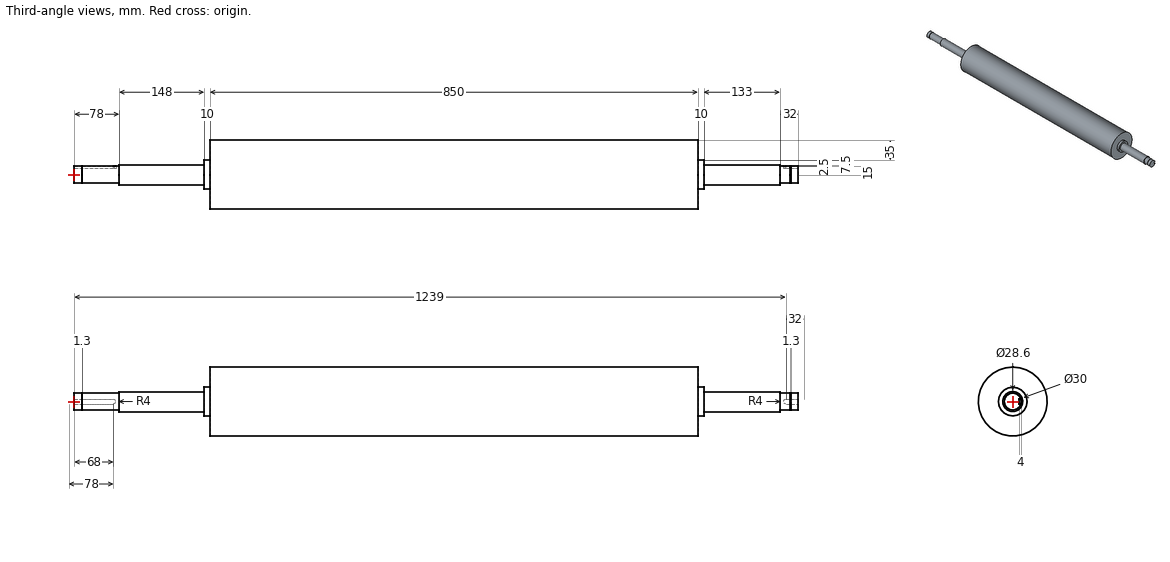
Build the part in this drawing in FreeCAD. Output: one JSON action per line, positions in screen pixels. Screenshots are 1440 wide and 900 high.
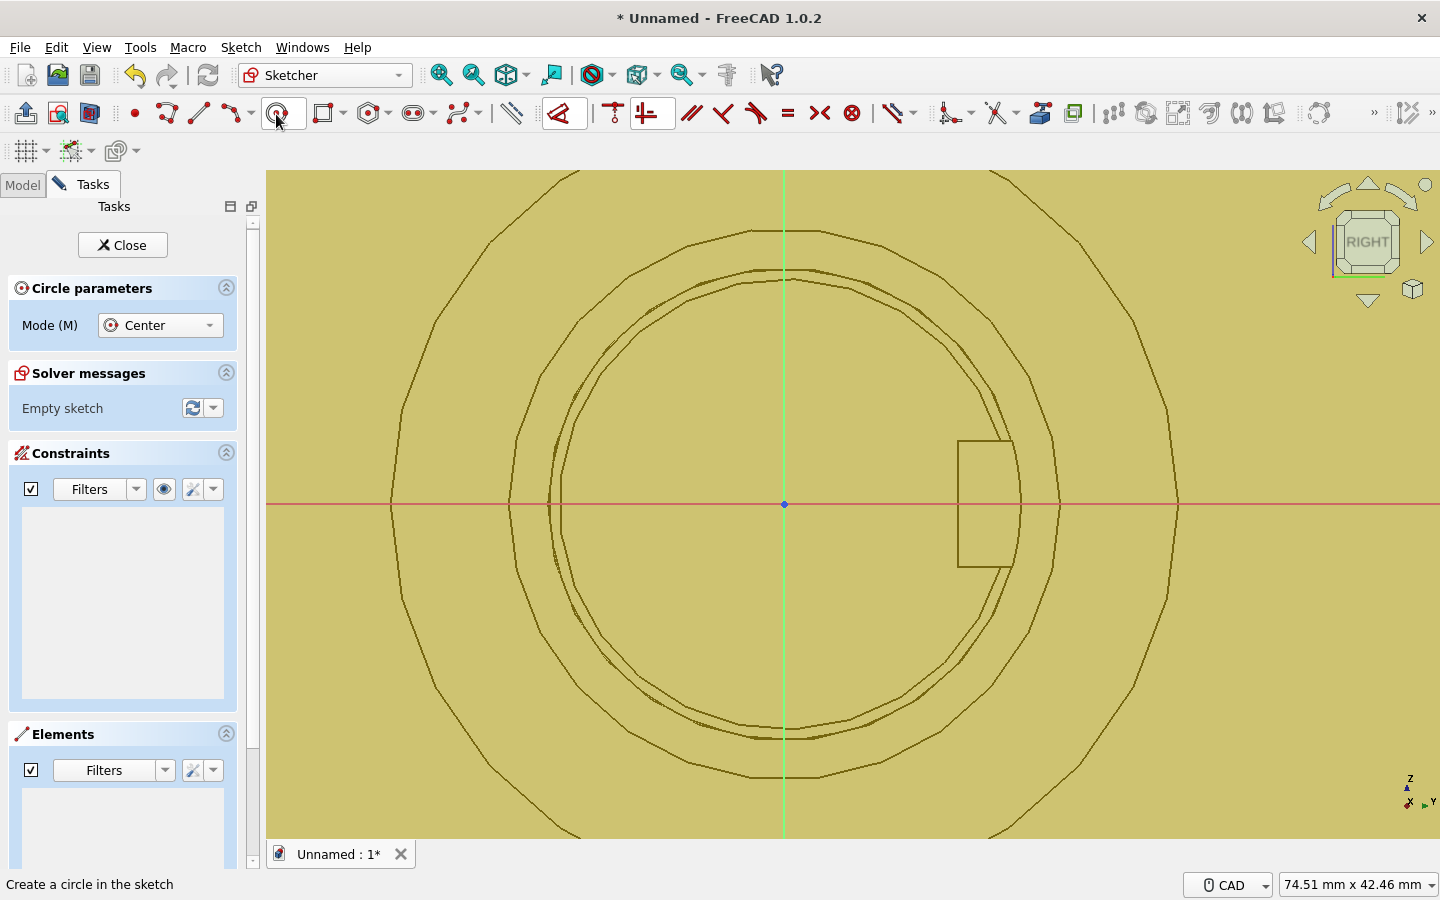
{"action": "left_click", "coordinate": [784, 504]}
{"action": "mouse_move", "coordinate": [952, 337]}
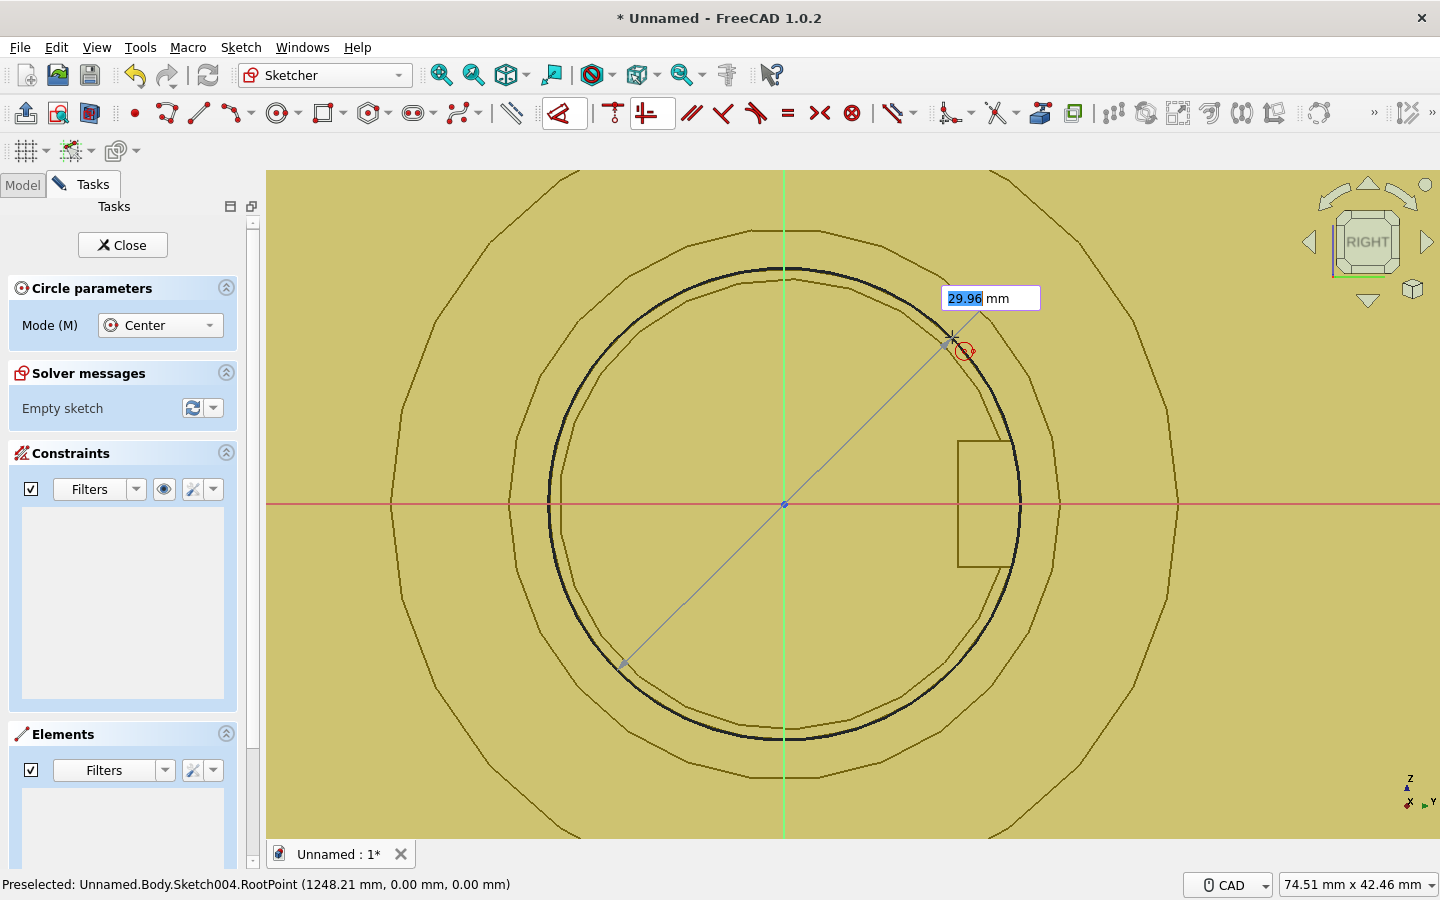
{"action": "type", "text": "30"}
{"action": "key", "text": "Return"}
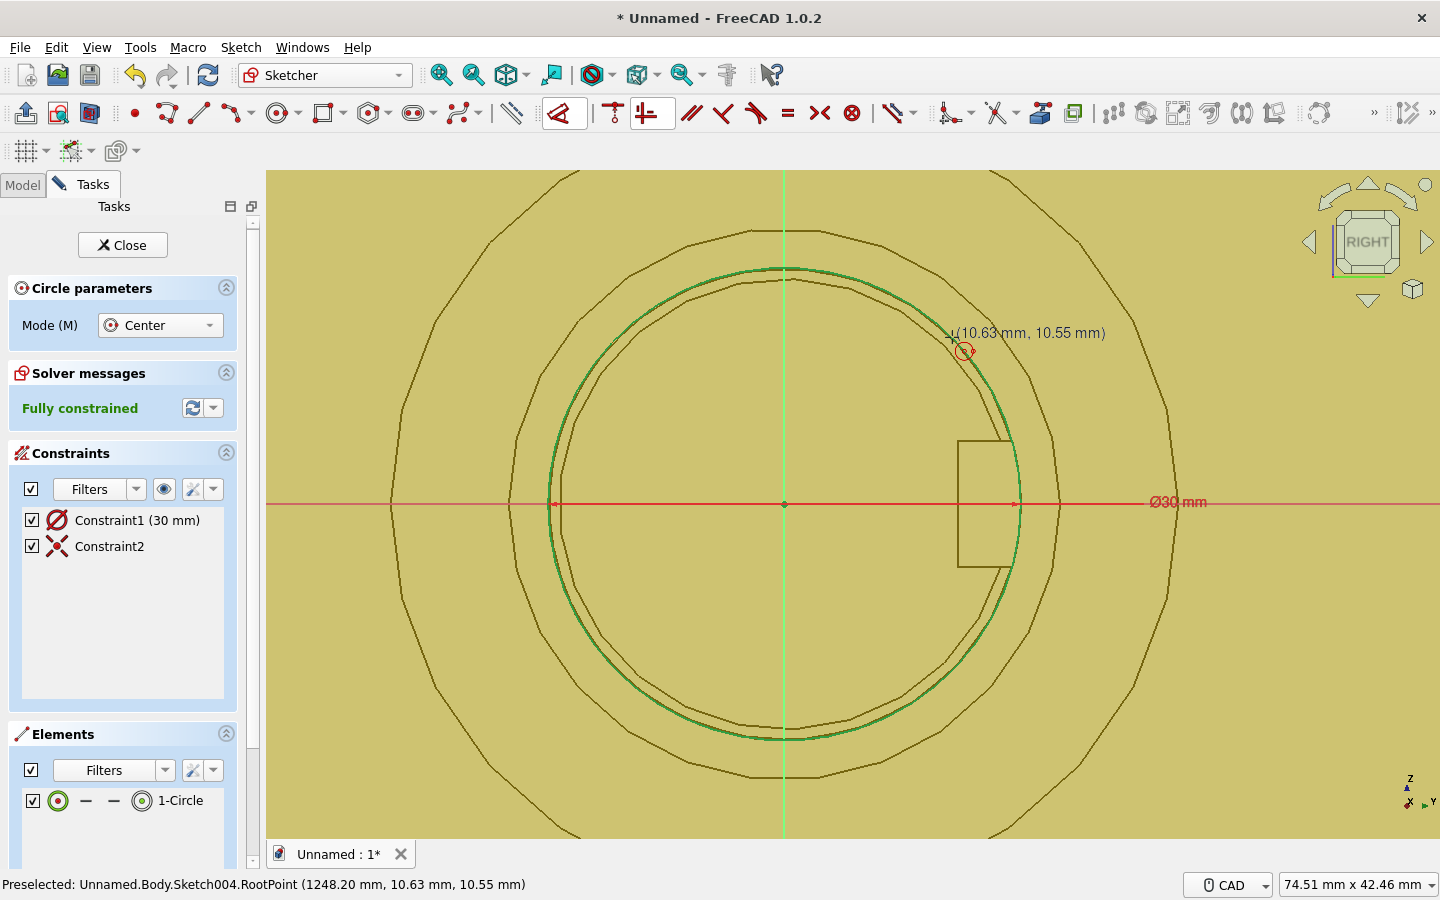
{"action": "left_click", "coordinate": [784, 504]}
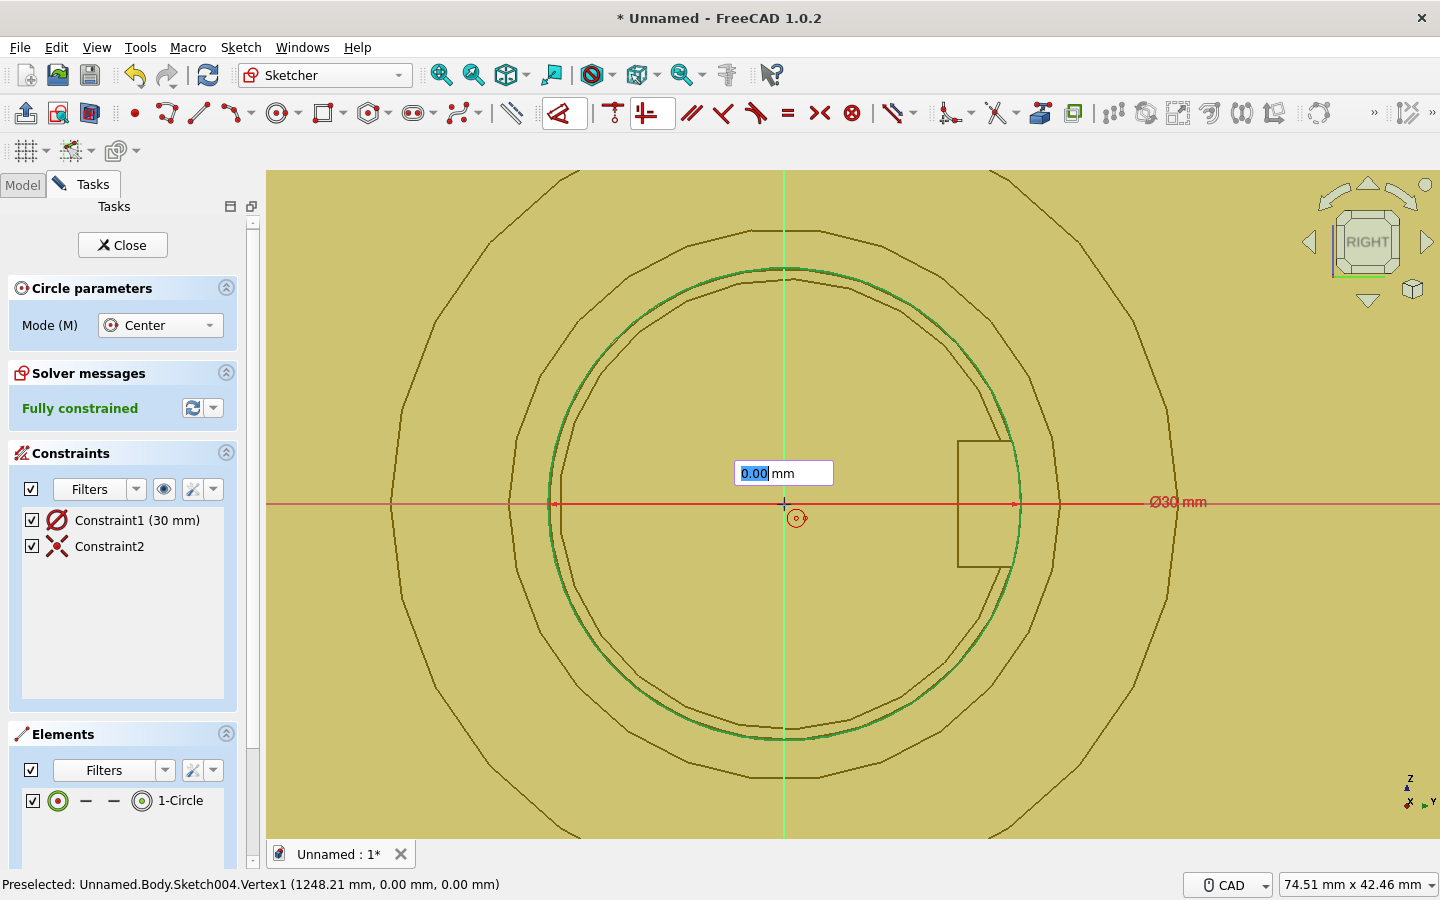
{"action": "scroll", "coordinate": [862, 293], "scroll_direction": "up", "scroll_amount": 2}
{"action": "mouse_move", "coordinate": [861, 292]}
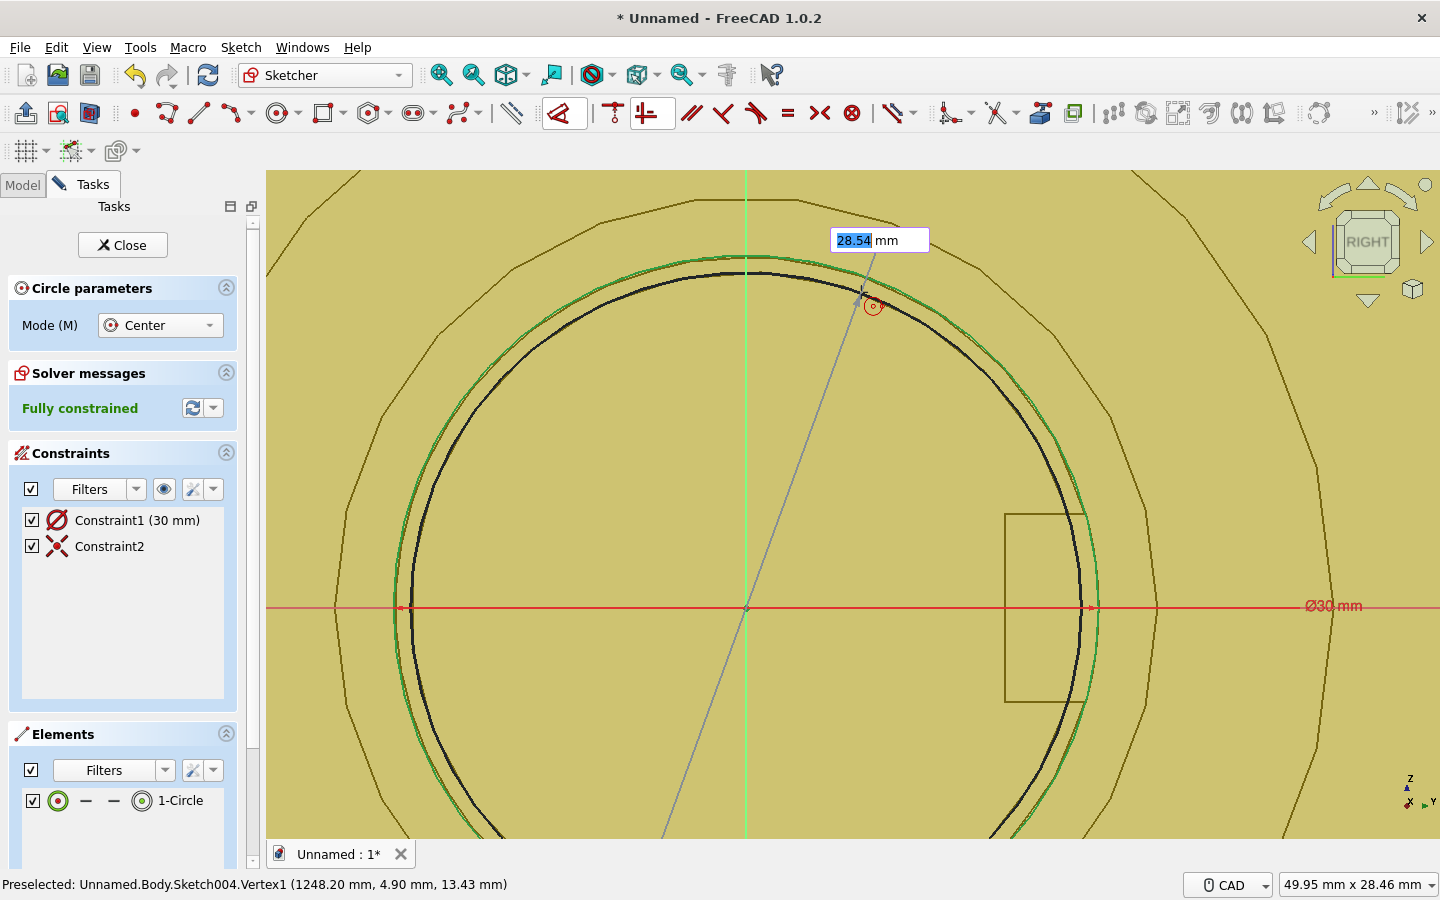
{"action": "type", "text": "28.6"}
{"action": "key", "text": "Return"}
{"action": "key", "text": "Escape"}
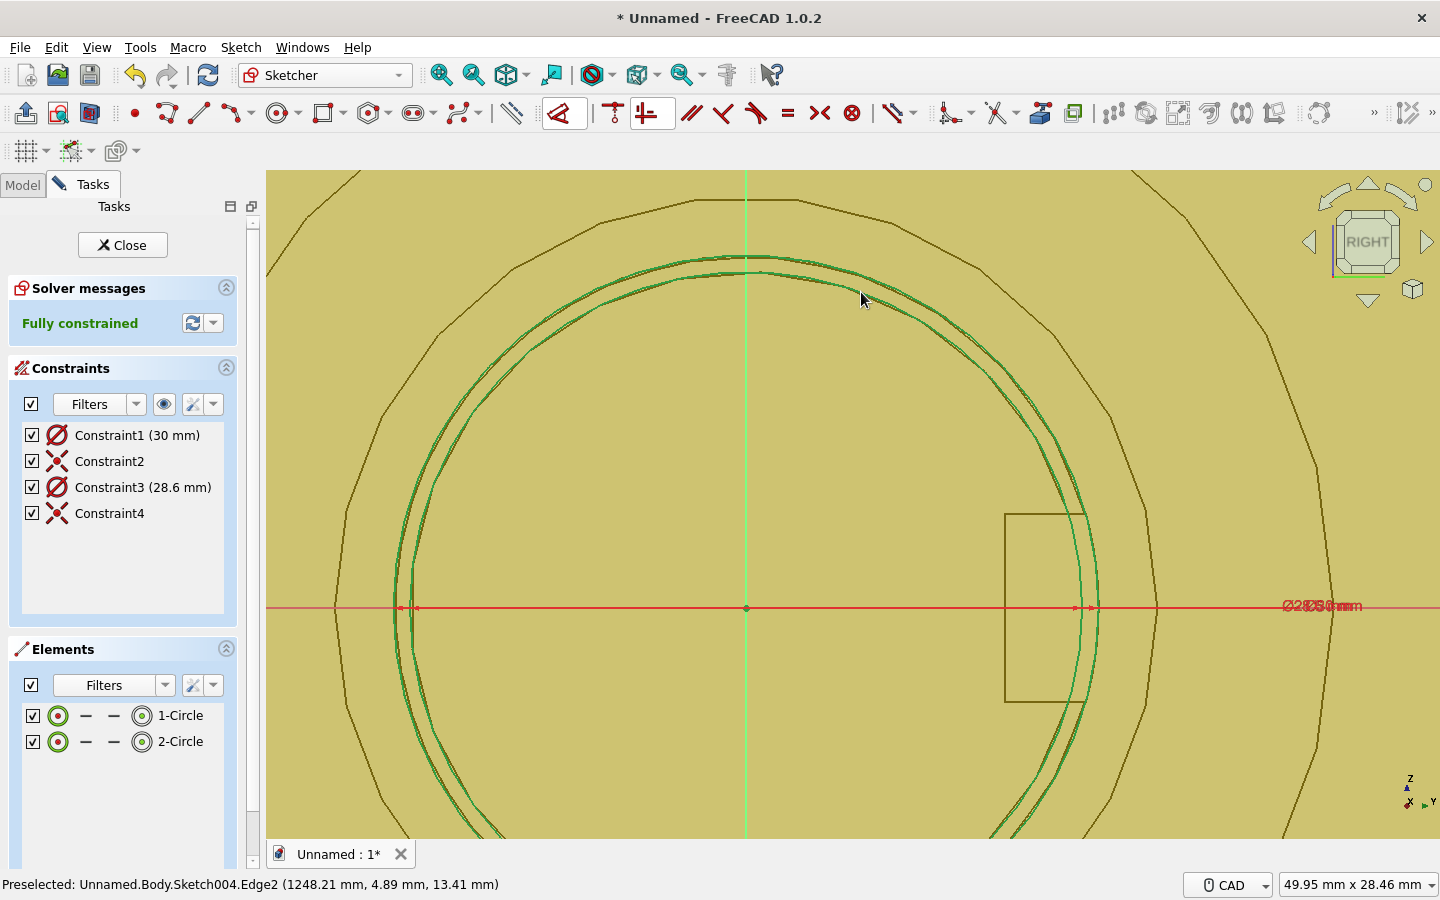
{"action": "left_click", "coordinate": [123, 245]}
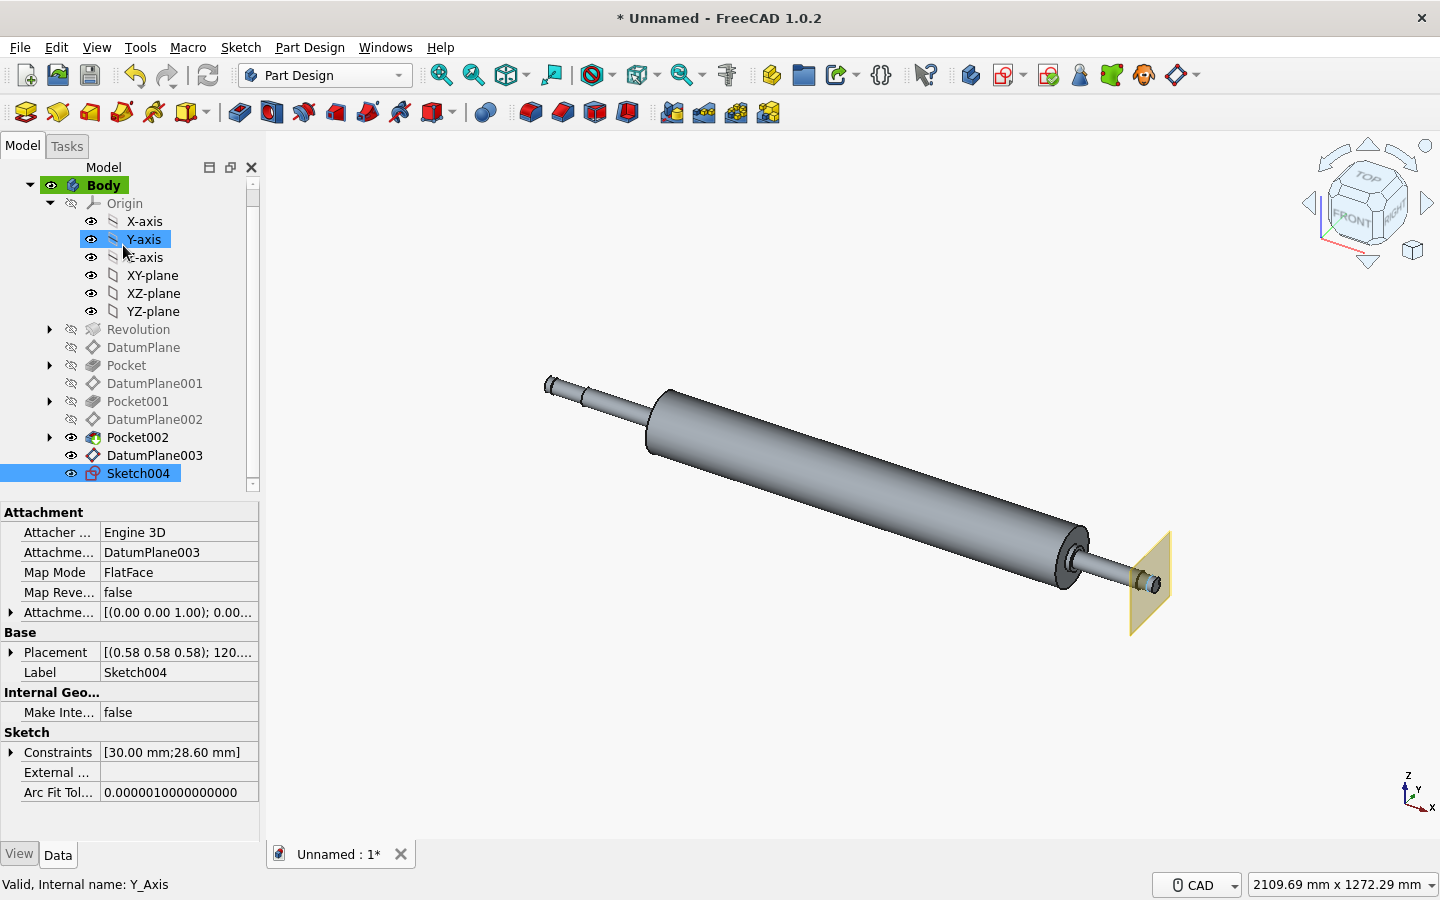
{"action": "left_click", "coordinate": [240, 112]}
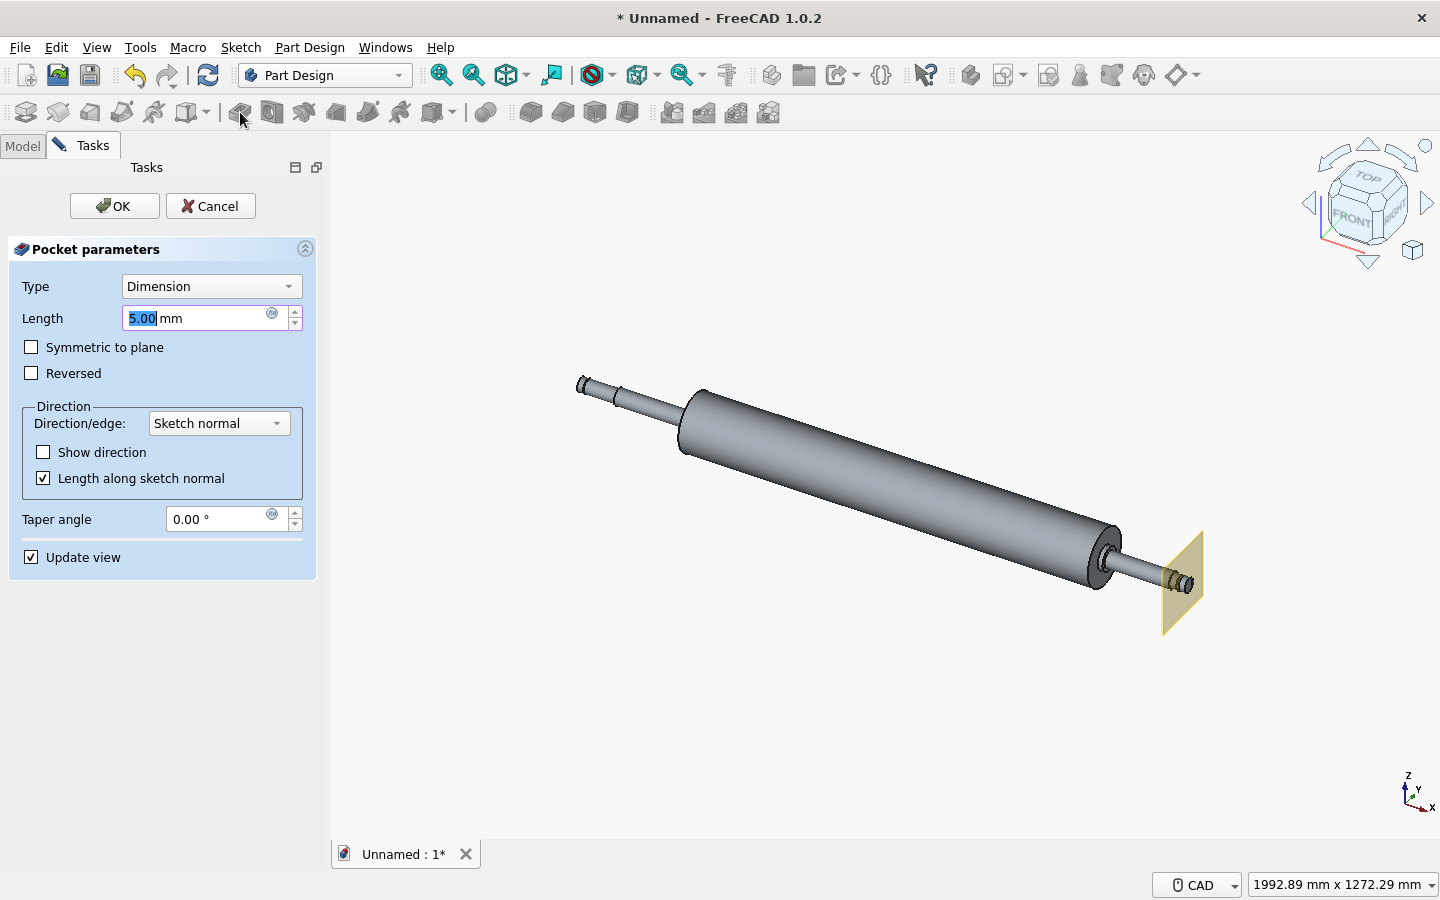
{"action": "type", "text": "1.3"}
{"action": "key", "text": "Tab"}